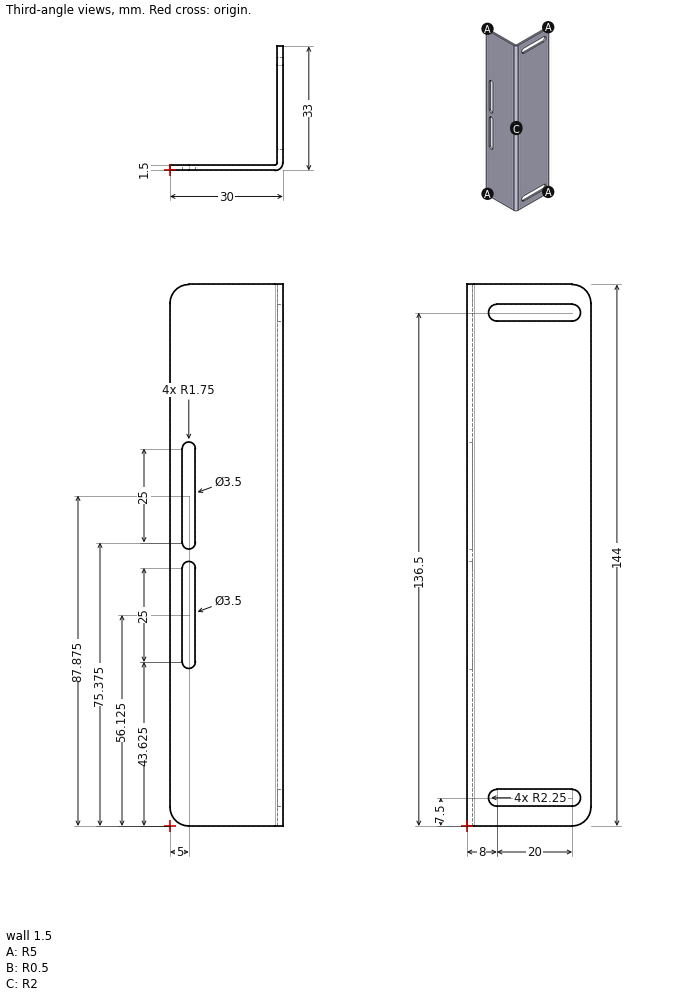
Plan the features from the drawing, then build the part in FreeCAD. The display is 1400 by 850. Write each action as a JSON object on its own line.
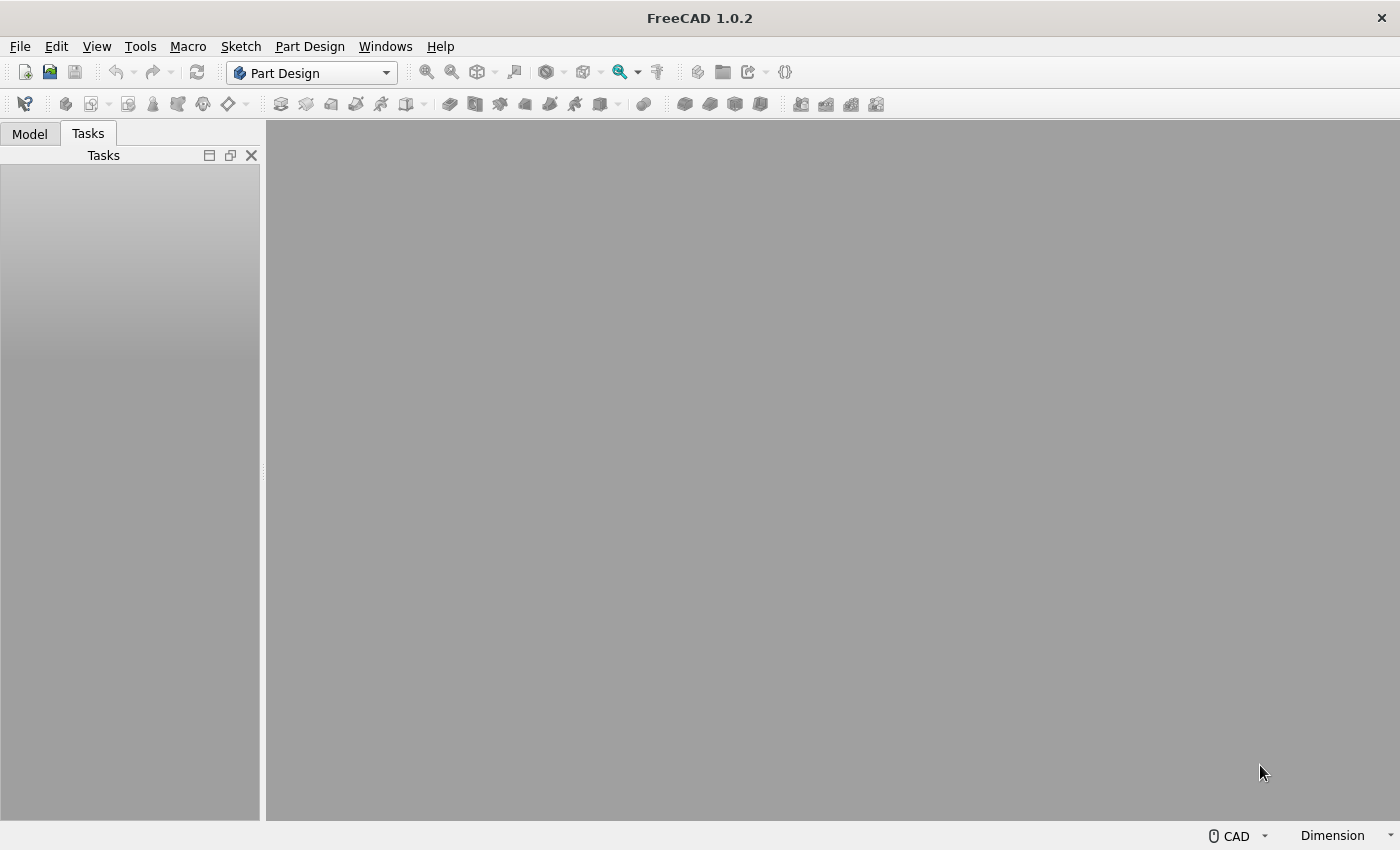
{"action": "left_click", "coordinate": [25, 72]}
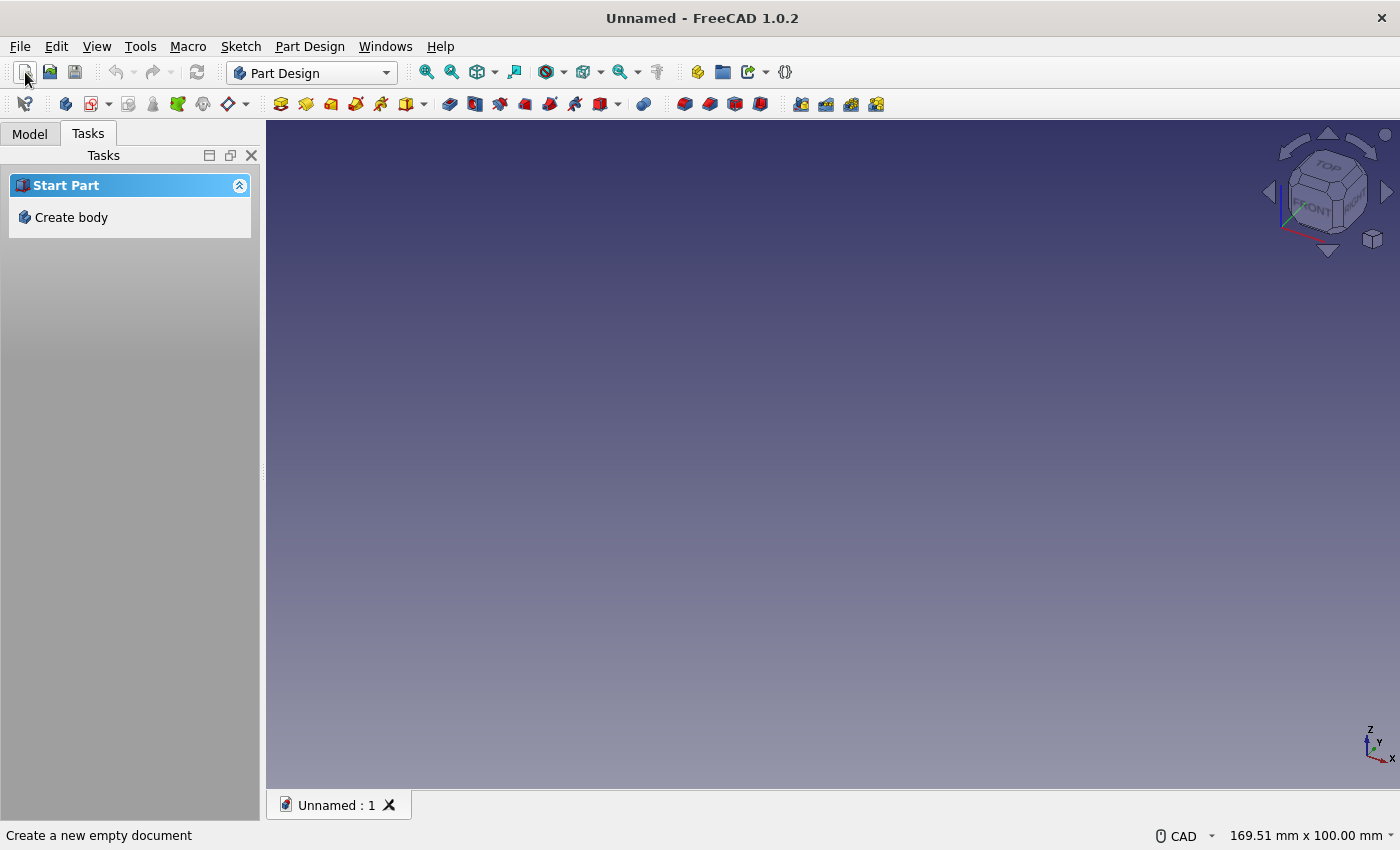
{"action": "left_click", "coordinate": [90, 104]}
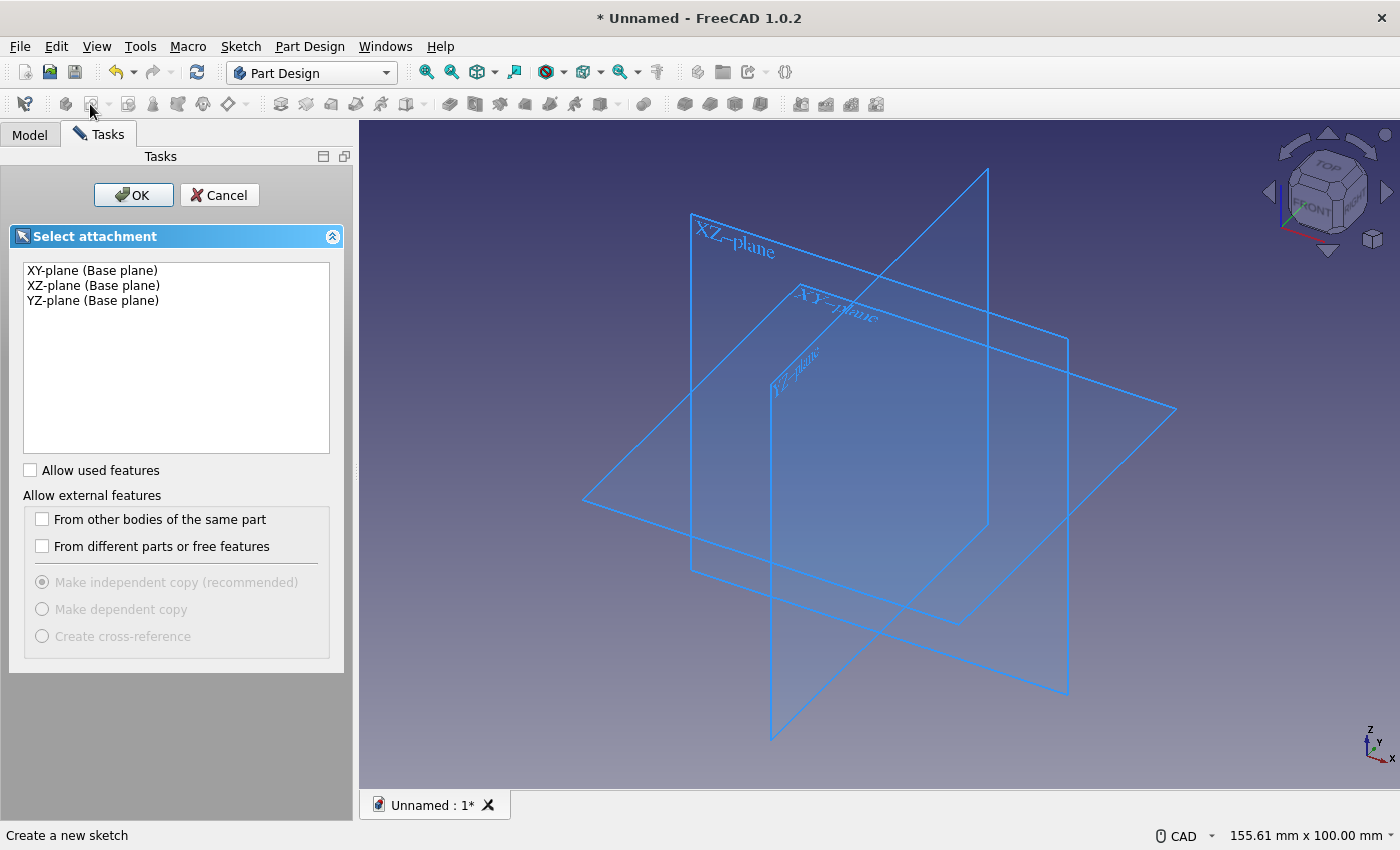
{"action": "left_click", "coordinate": [84, 270]}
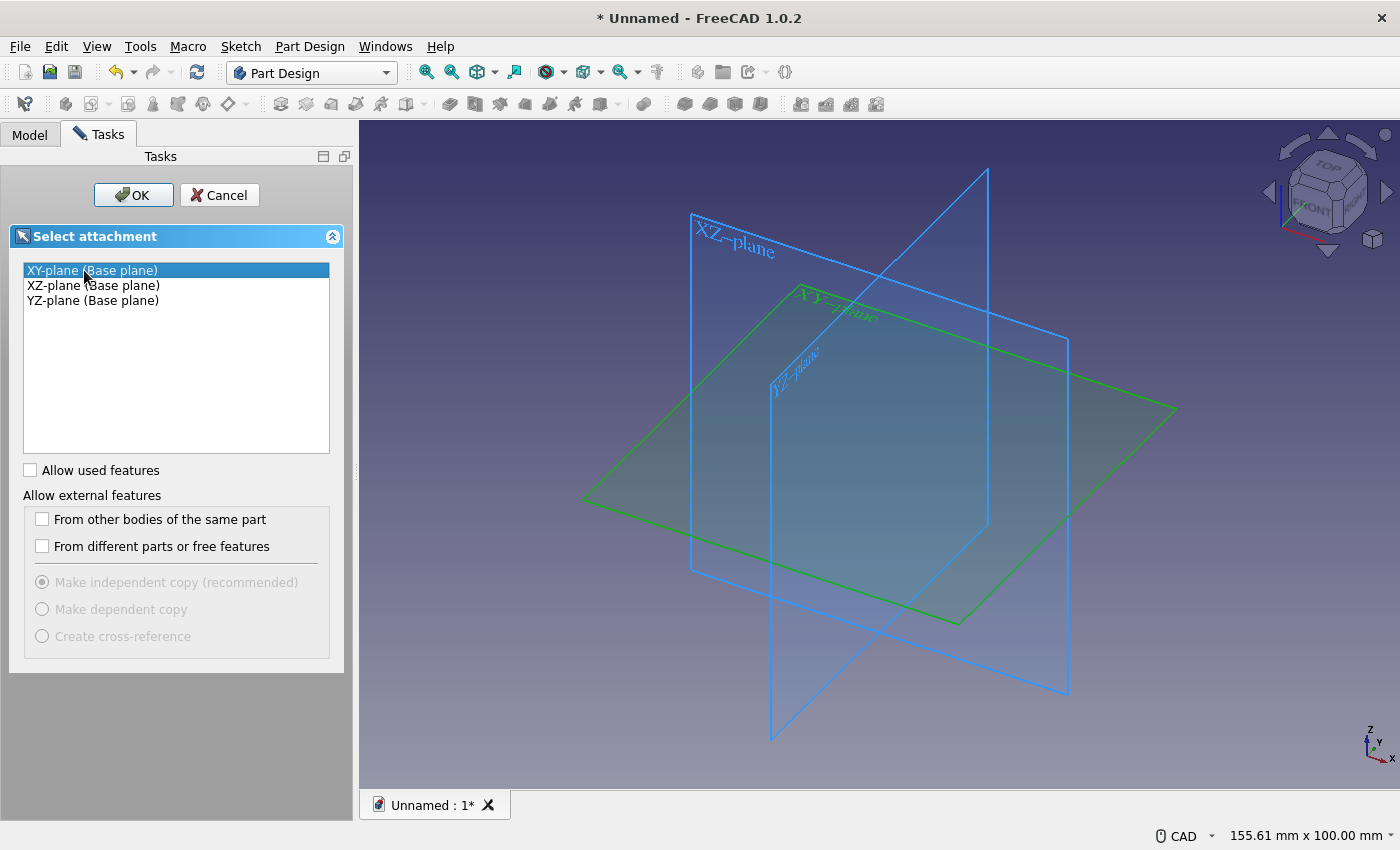
{"action": "left_click", "coordinate": [134, 195]}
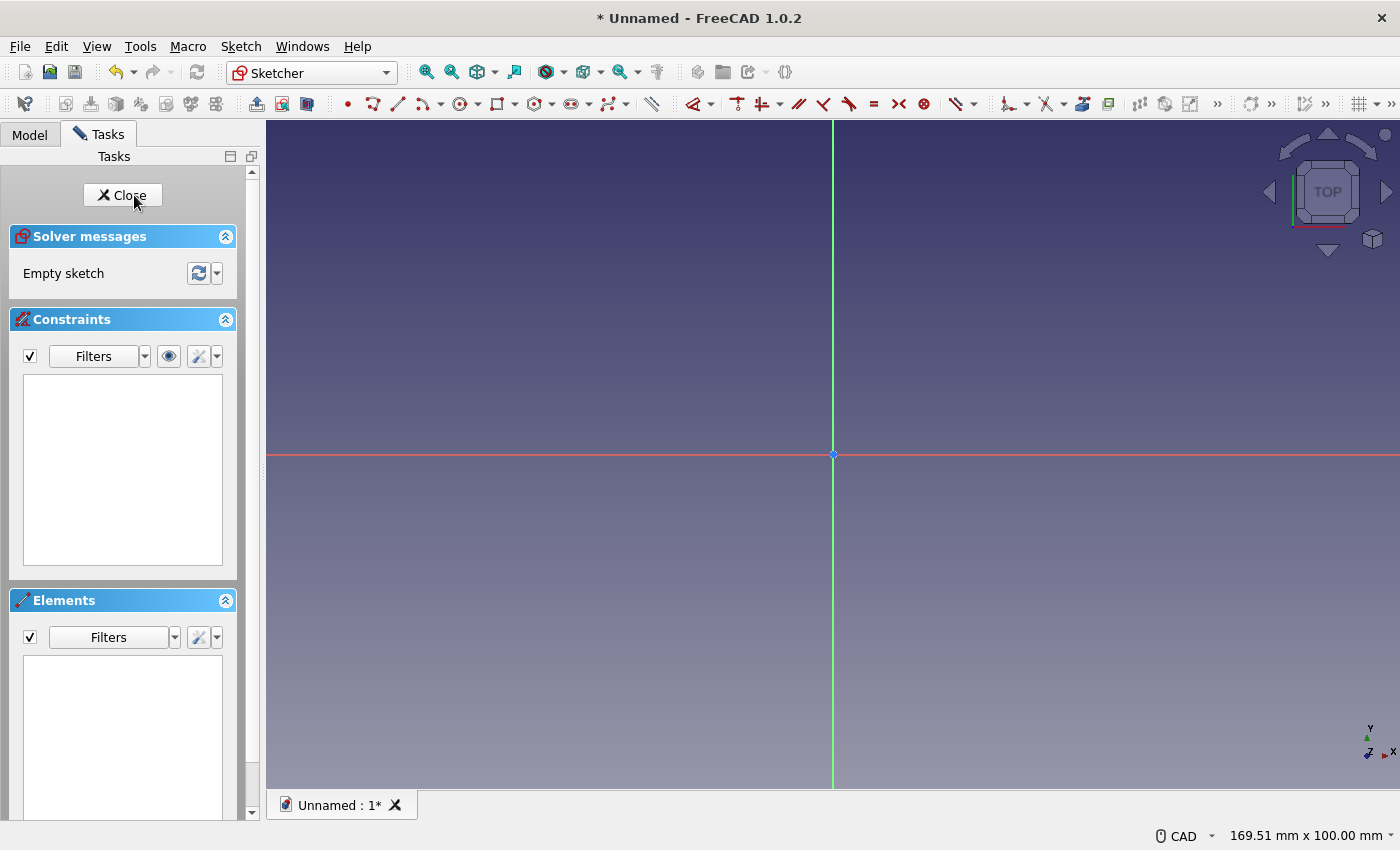
{"action": "scroll", "coordinate": [1139, 210], "scroll_direction": "up", "scroll_amount": 3}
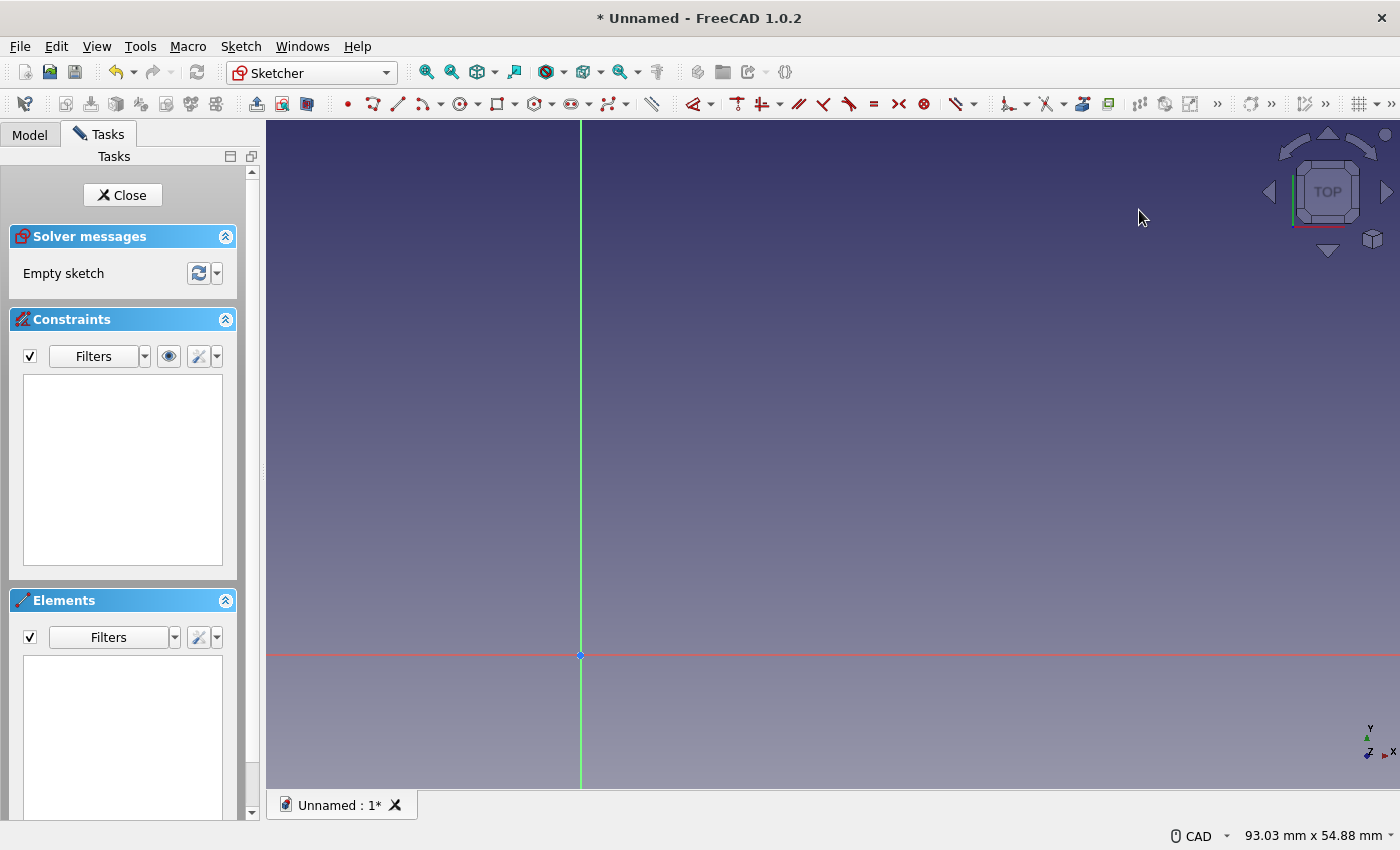
{"action": "left_click", "coordinate": [496, 104]}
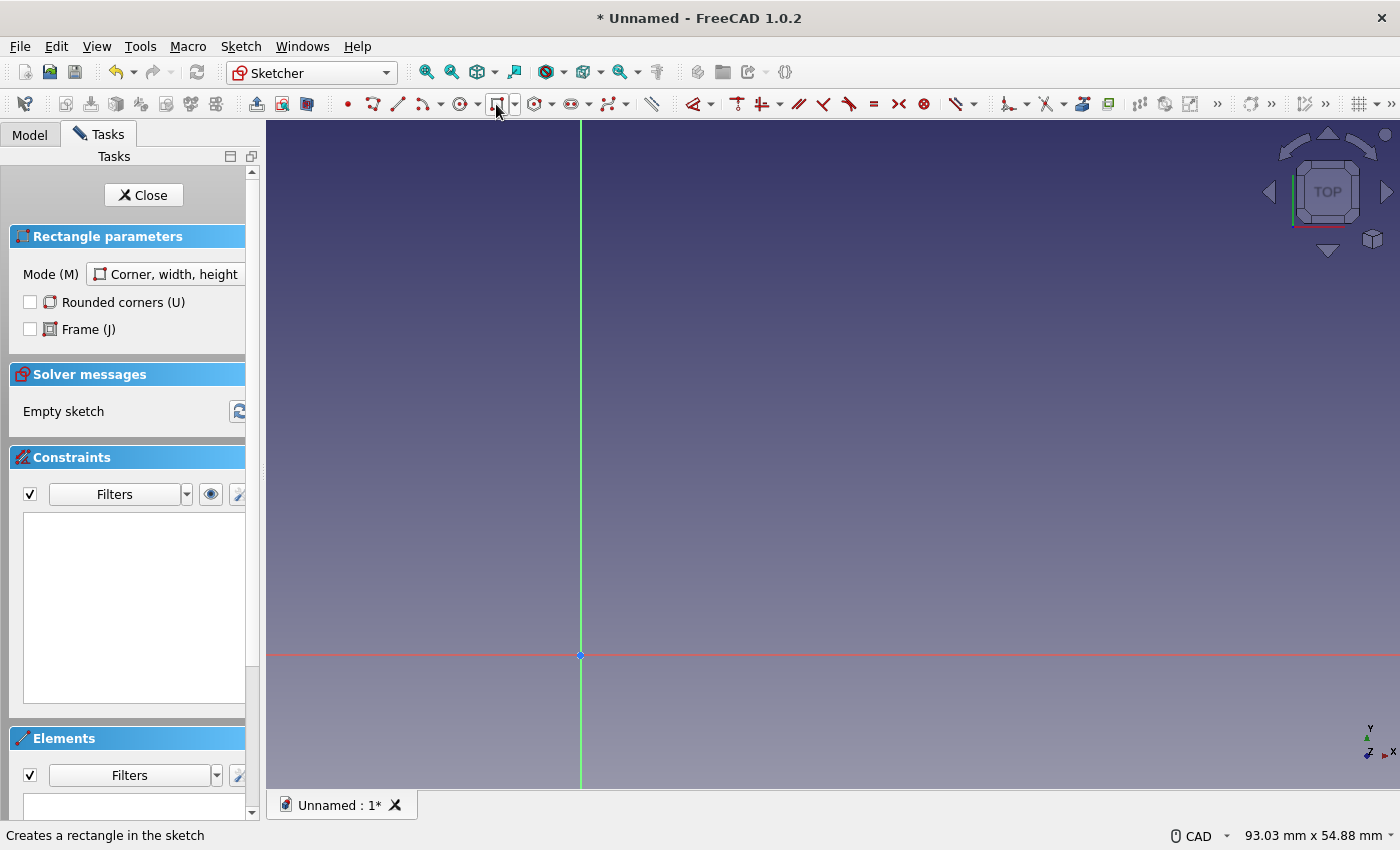
{"action": "left_click", "coordinate": [581, 655]}
{"action": "left_click", "coordinate": [946, 253]}
{"action": "key", "text": "Escape"}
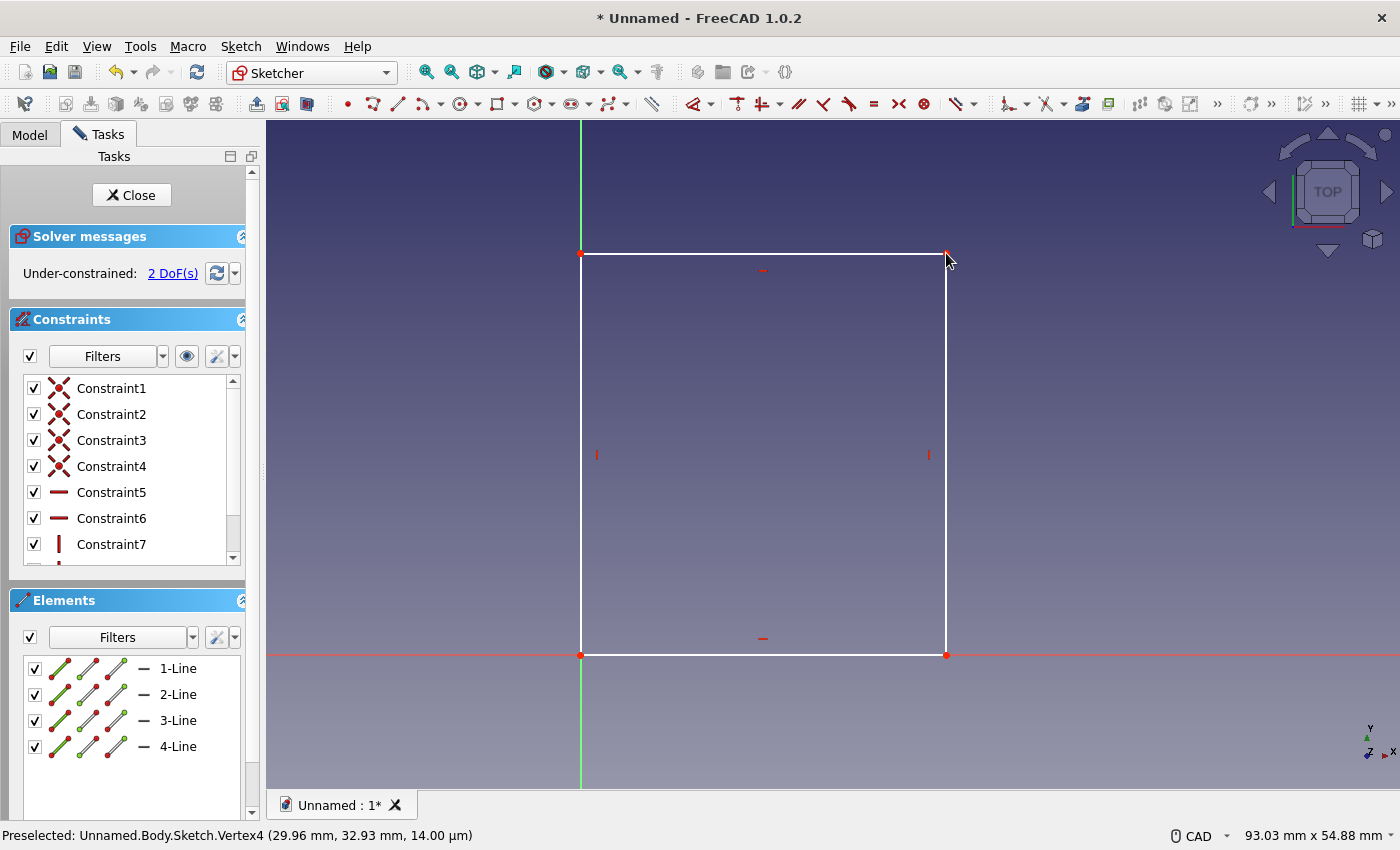
{"action": "left_click", "coordinate": [690, 655]}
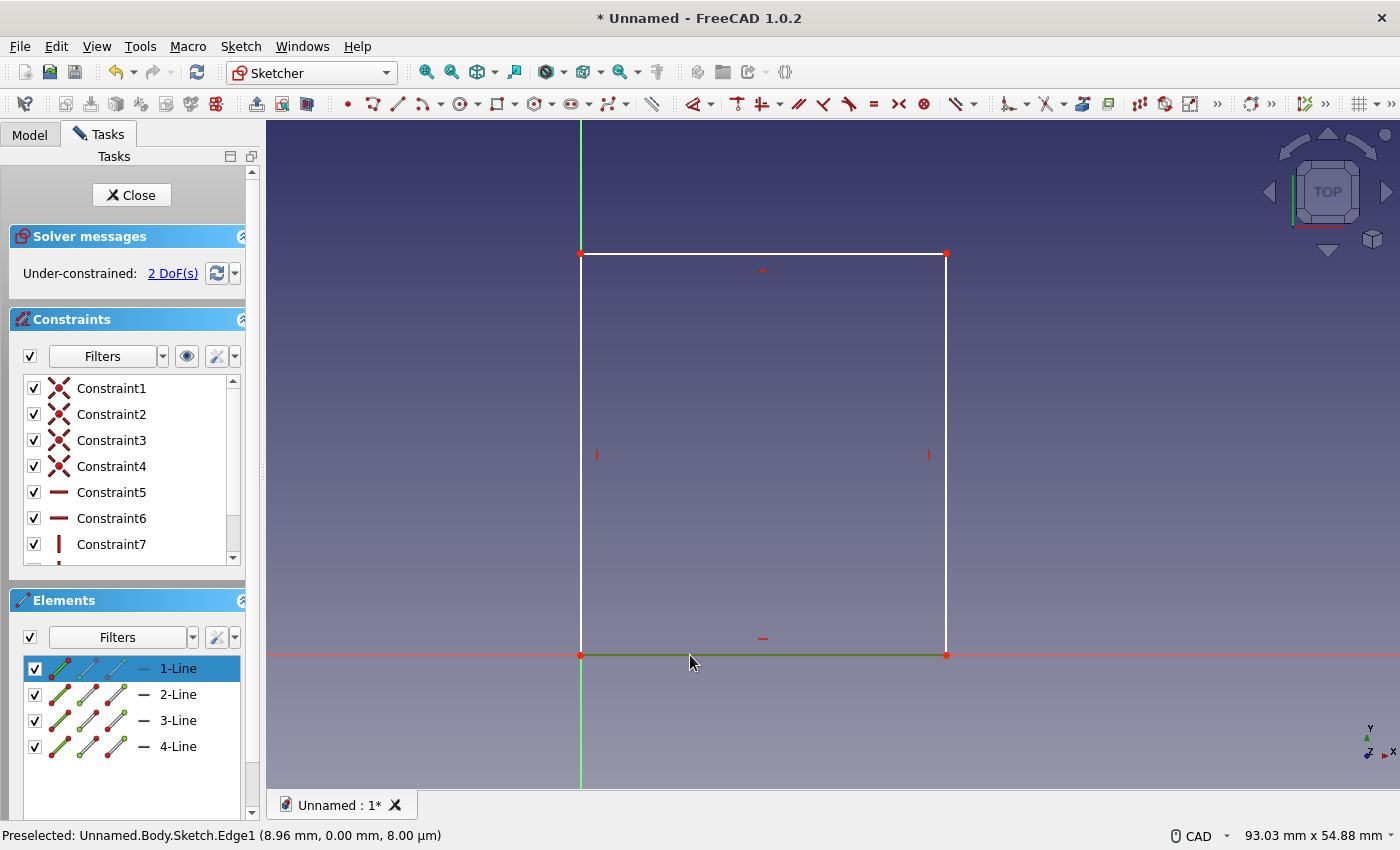
{"action": "left_click", "coordinate": [710, 104]}